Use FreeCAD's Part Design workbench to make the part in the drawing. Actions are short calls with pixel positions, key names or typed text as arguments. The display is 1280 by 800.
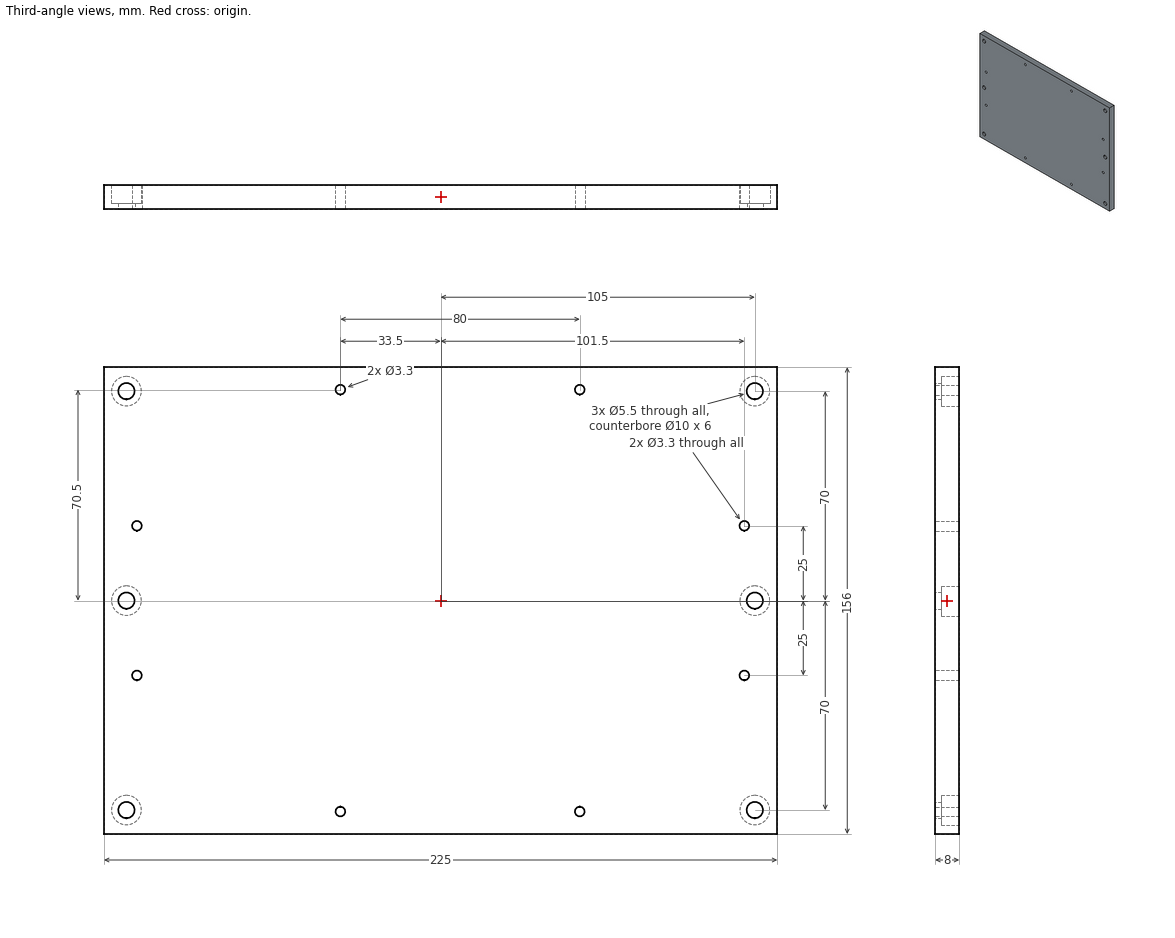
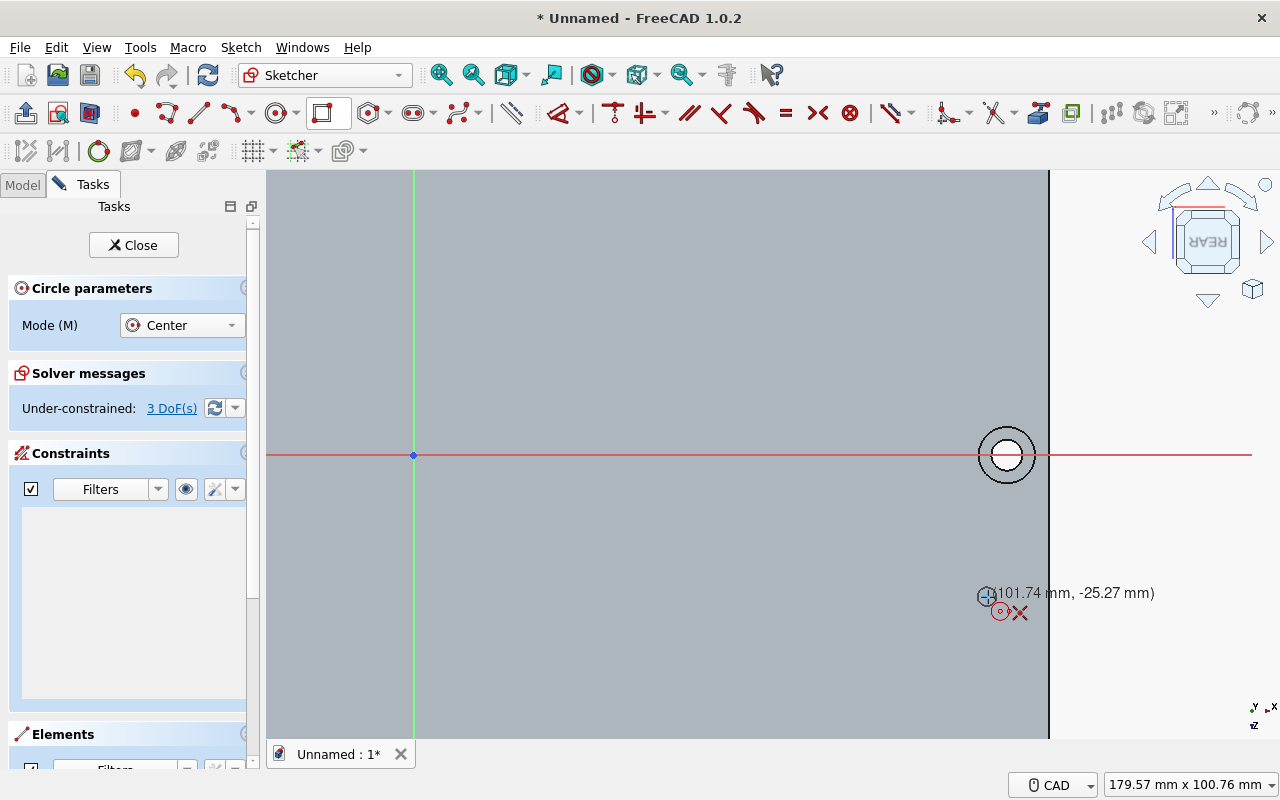
scroll(987, 314, up, 5)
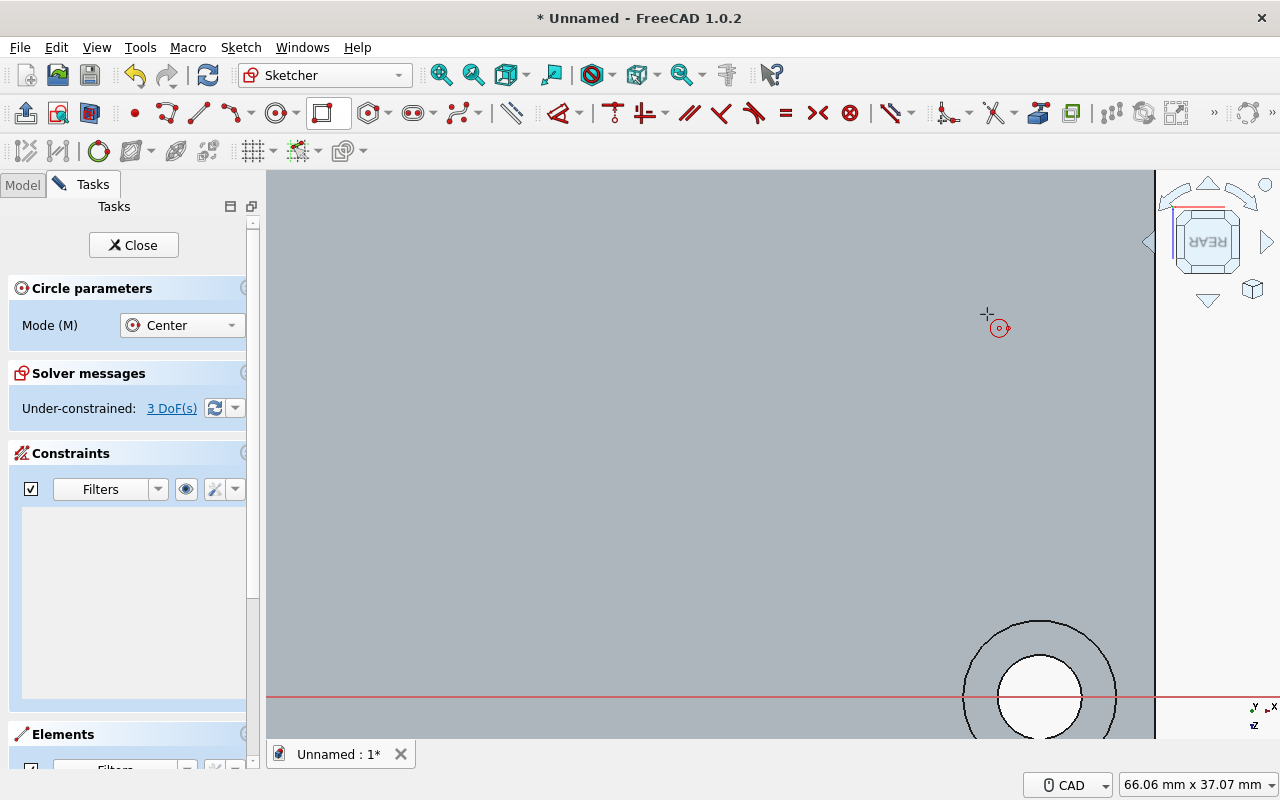
click(986, 313)
click(1004, 296)
key(Escape)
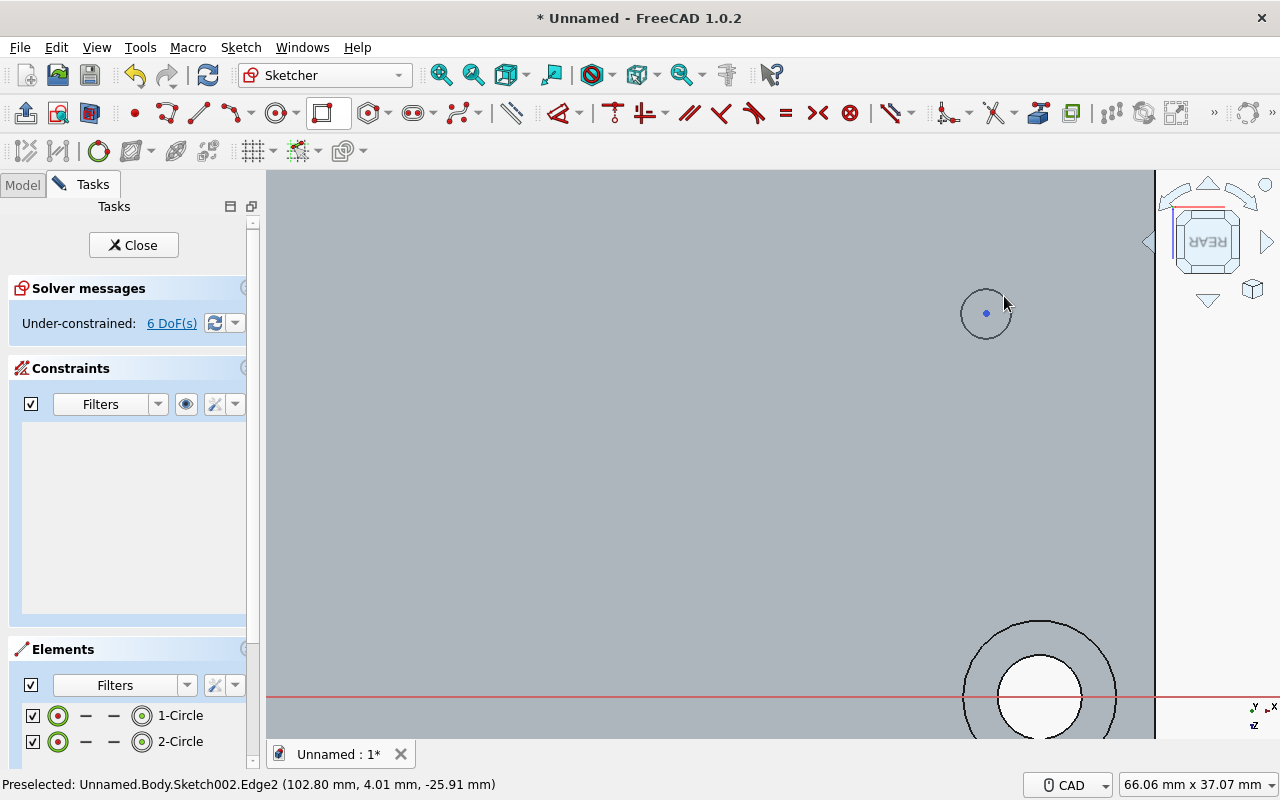
scroll(987, 313, down, 5)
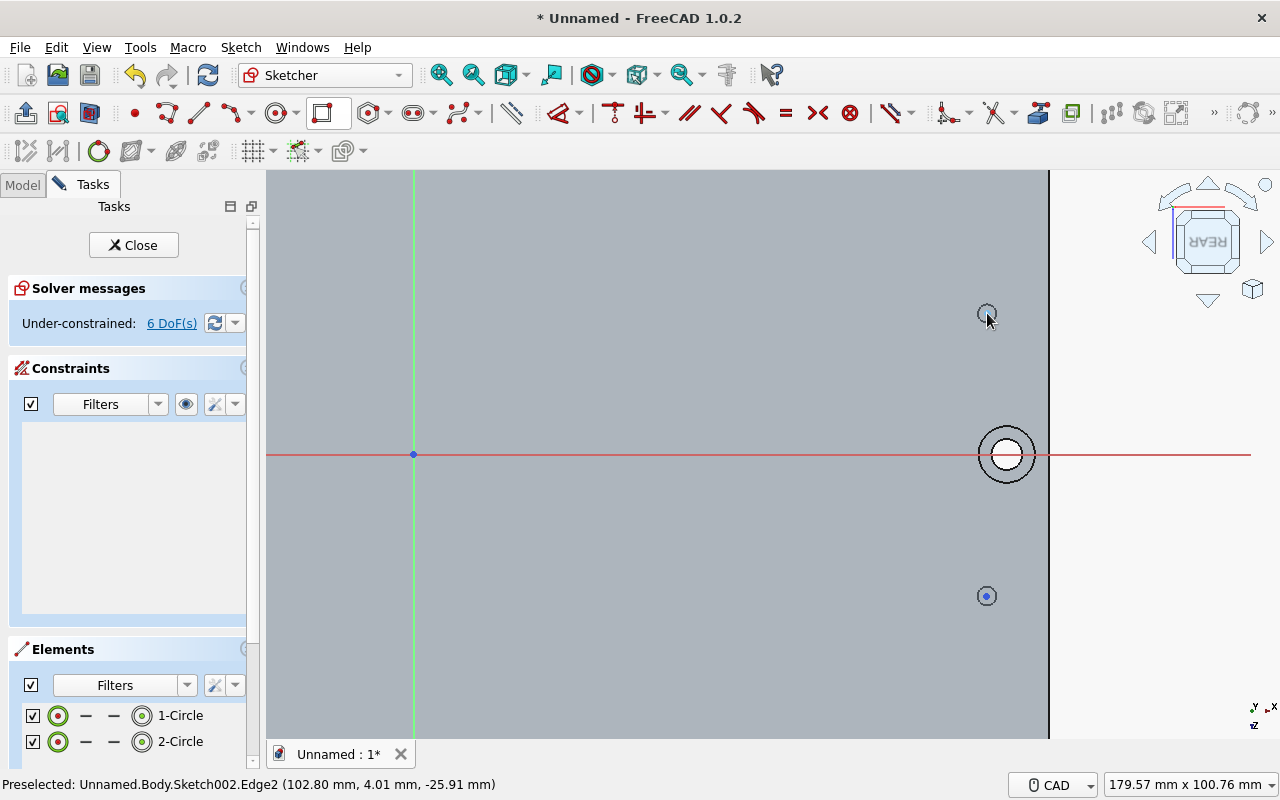
scroll(994, 589, up, 2)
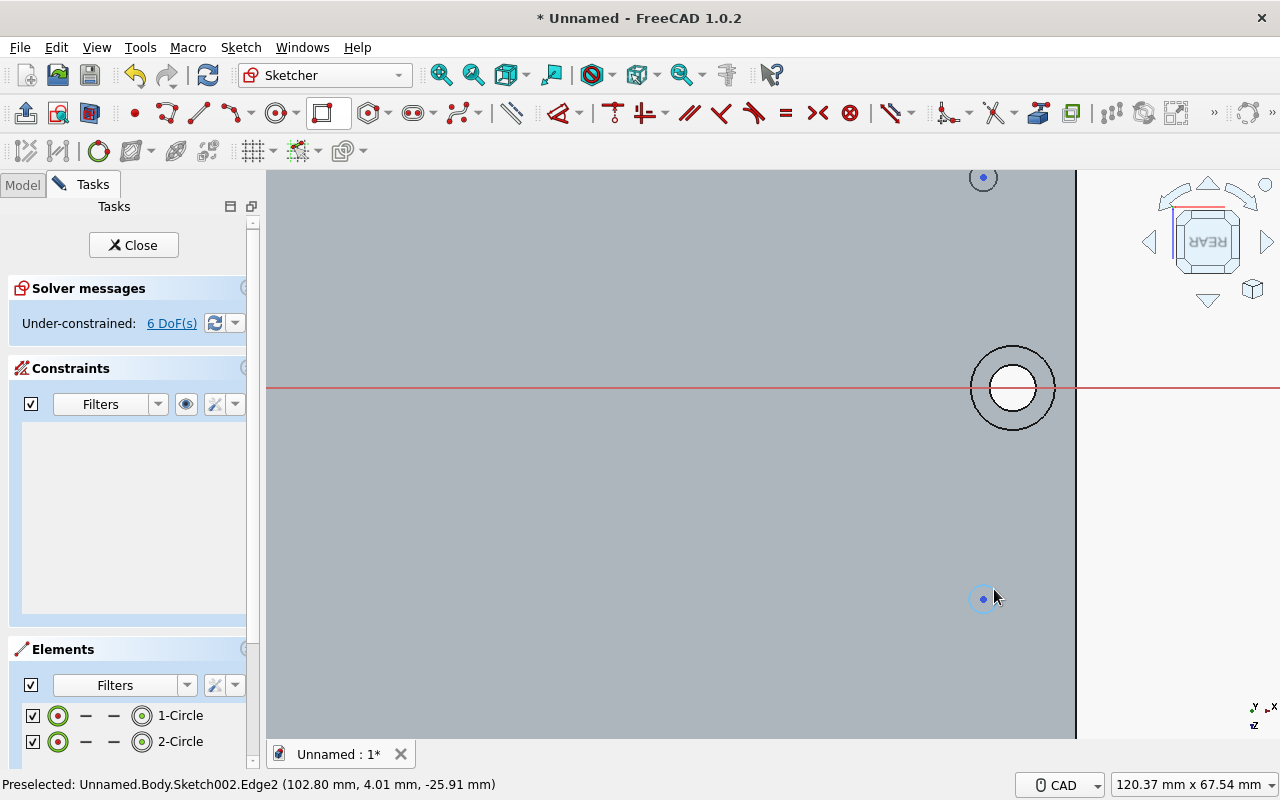
click(993, 589)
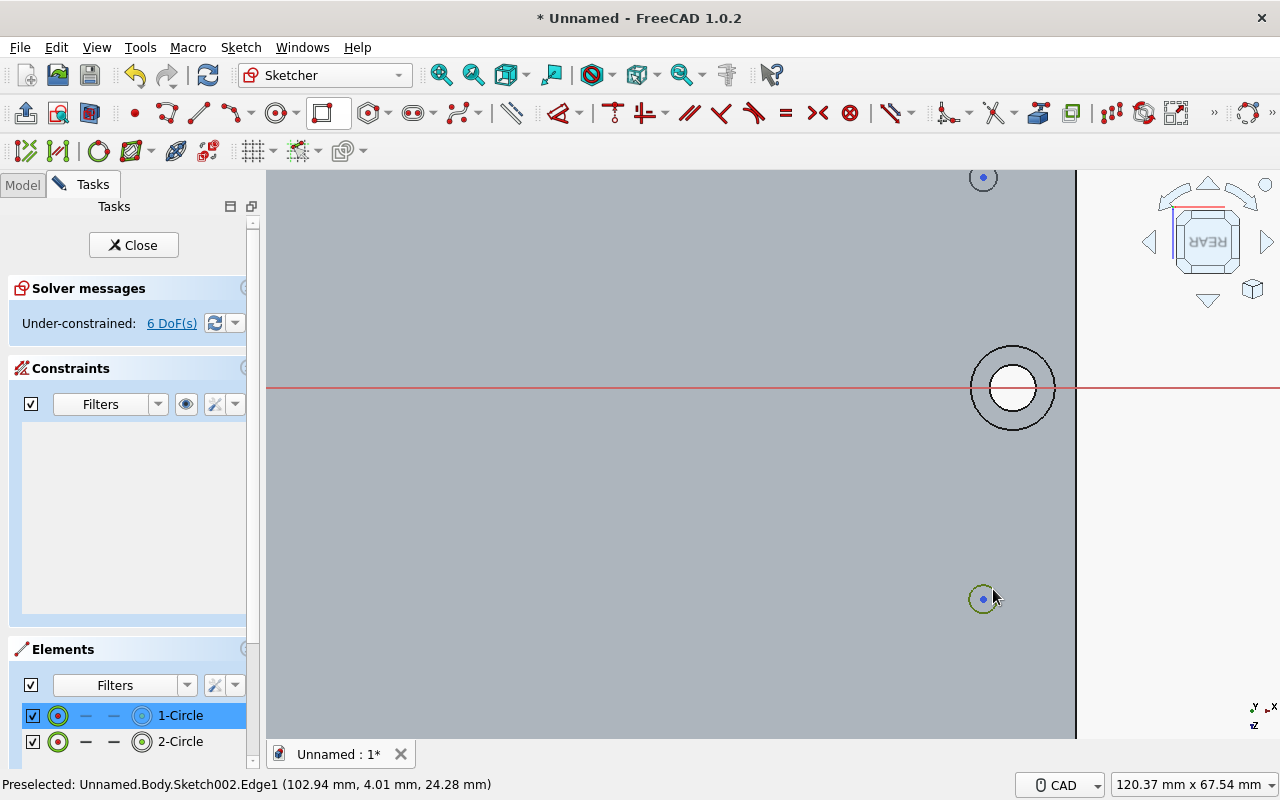
scroll(993, 590, down, 2)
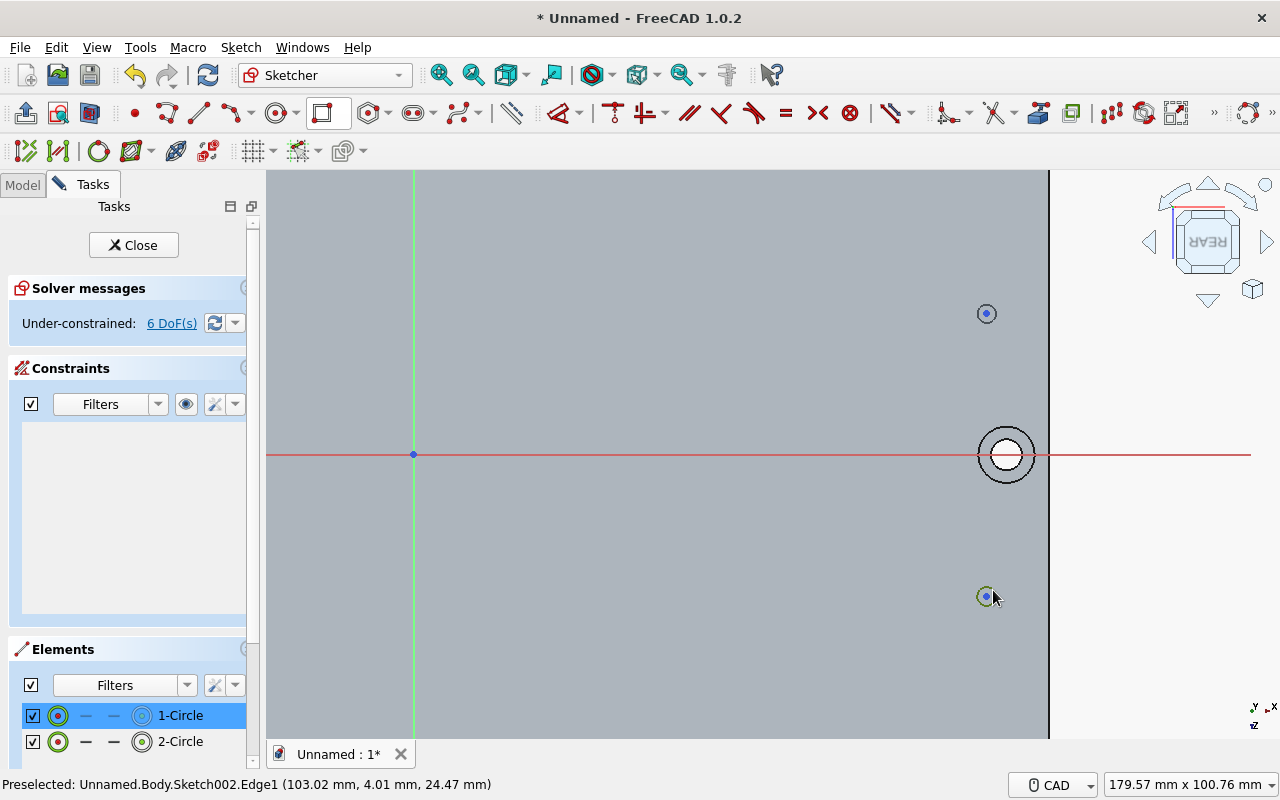
scroll(993, 307, up, 3)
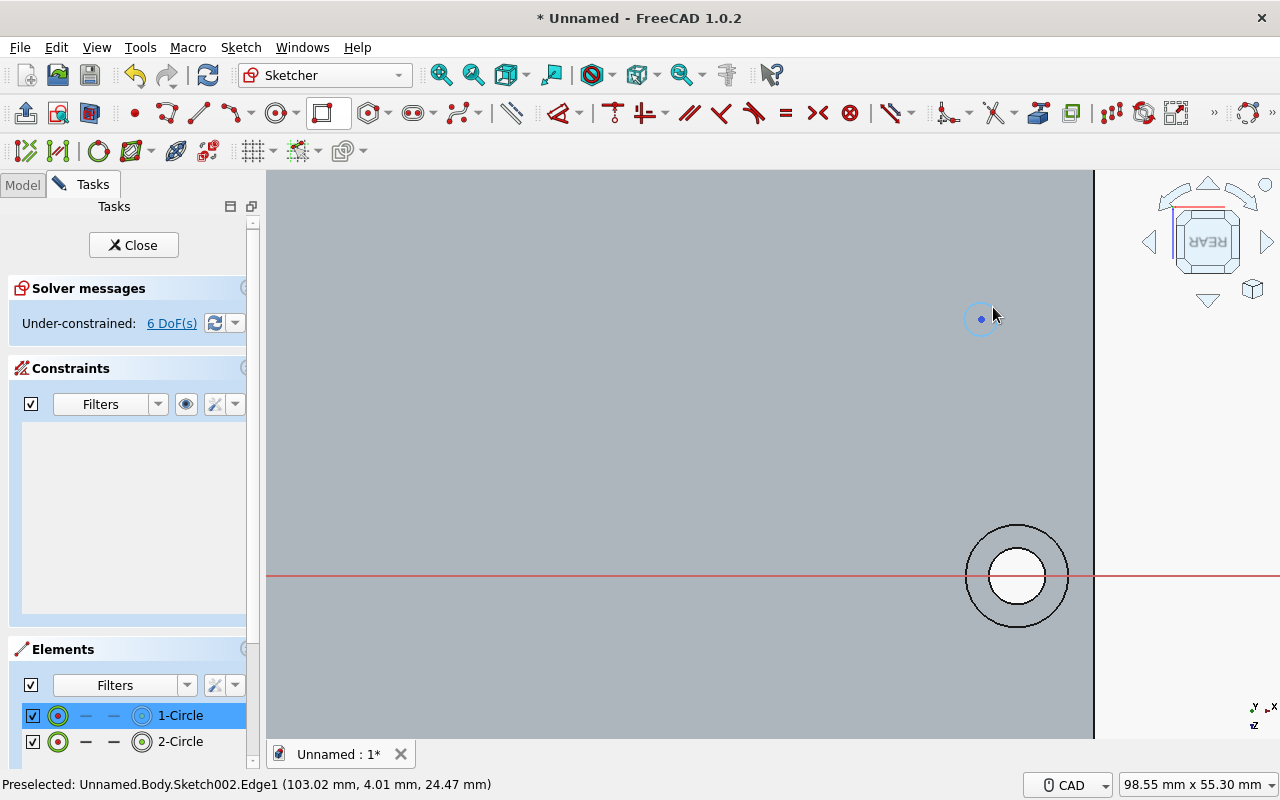
click(993, 308)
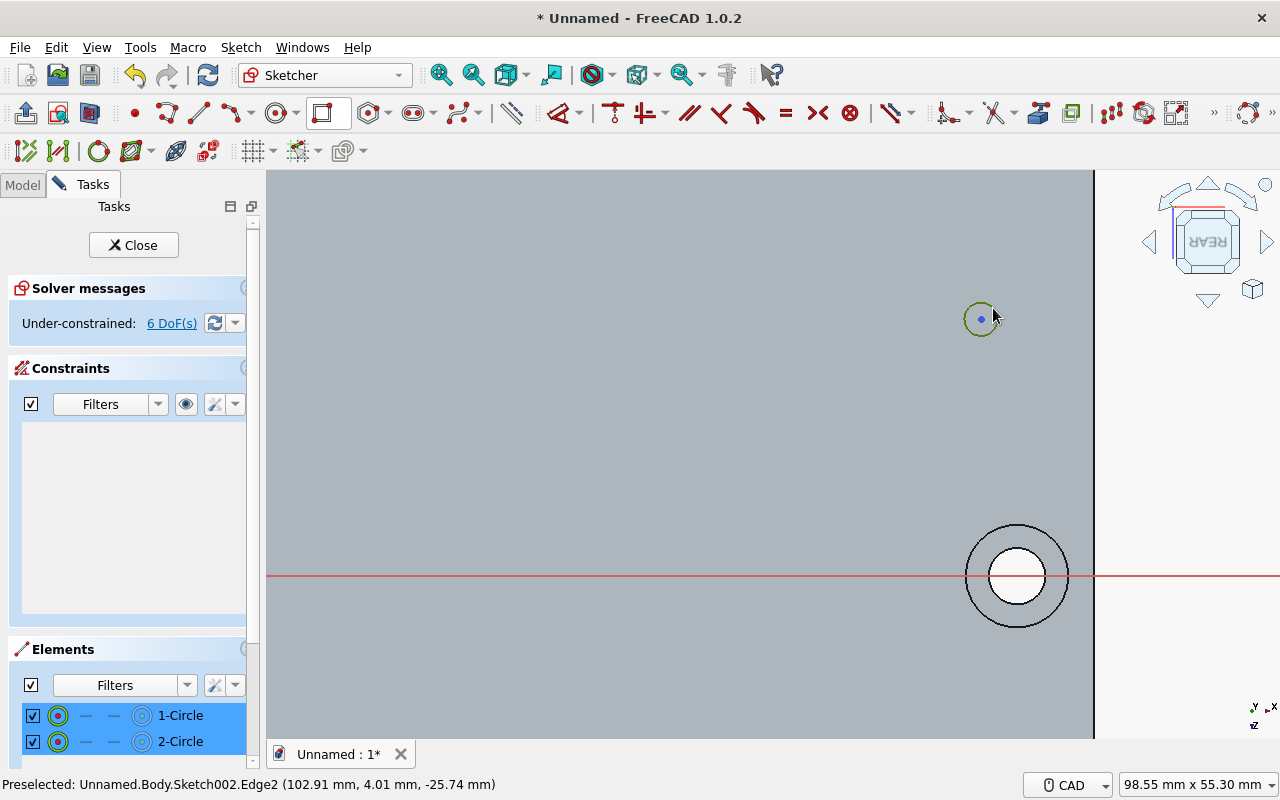
click(786, 114)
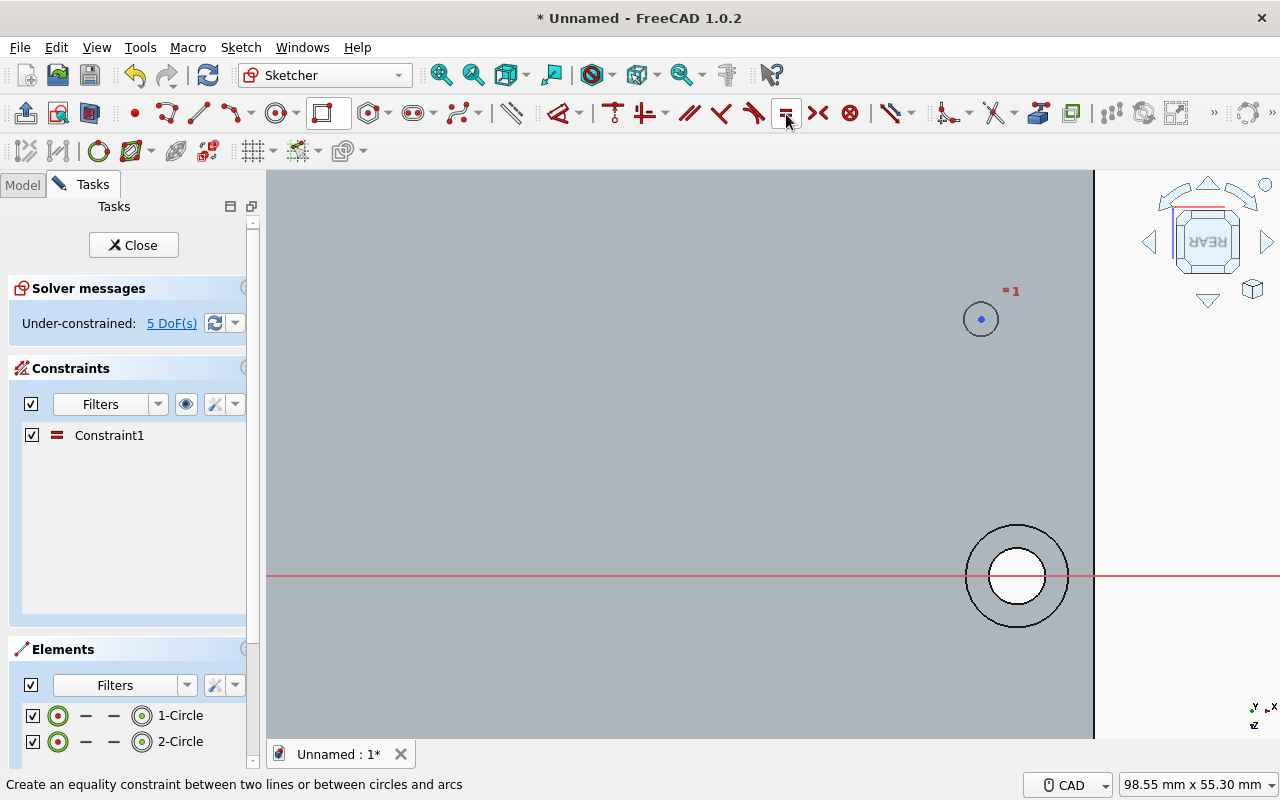
scroll(993, 307, down, 3)